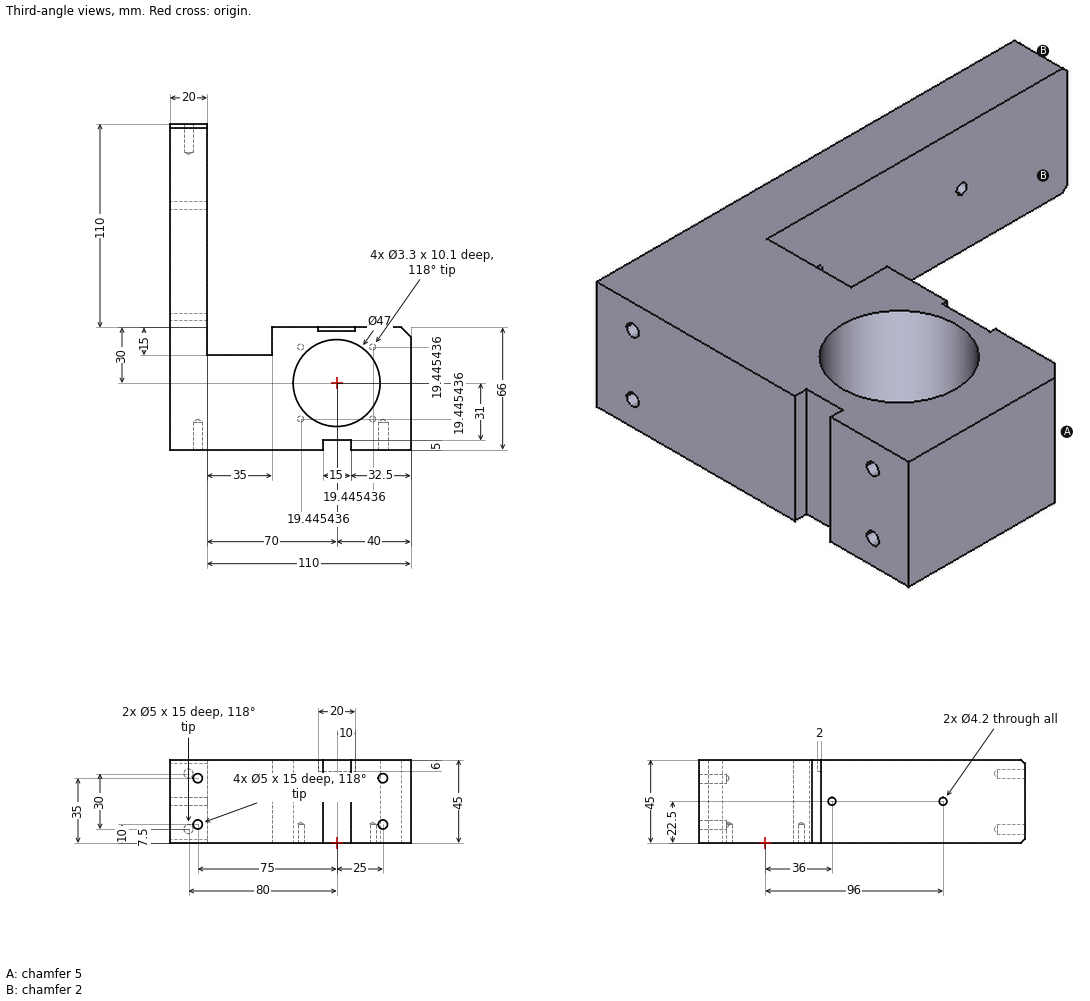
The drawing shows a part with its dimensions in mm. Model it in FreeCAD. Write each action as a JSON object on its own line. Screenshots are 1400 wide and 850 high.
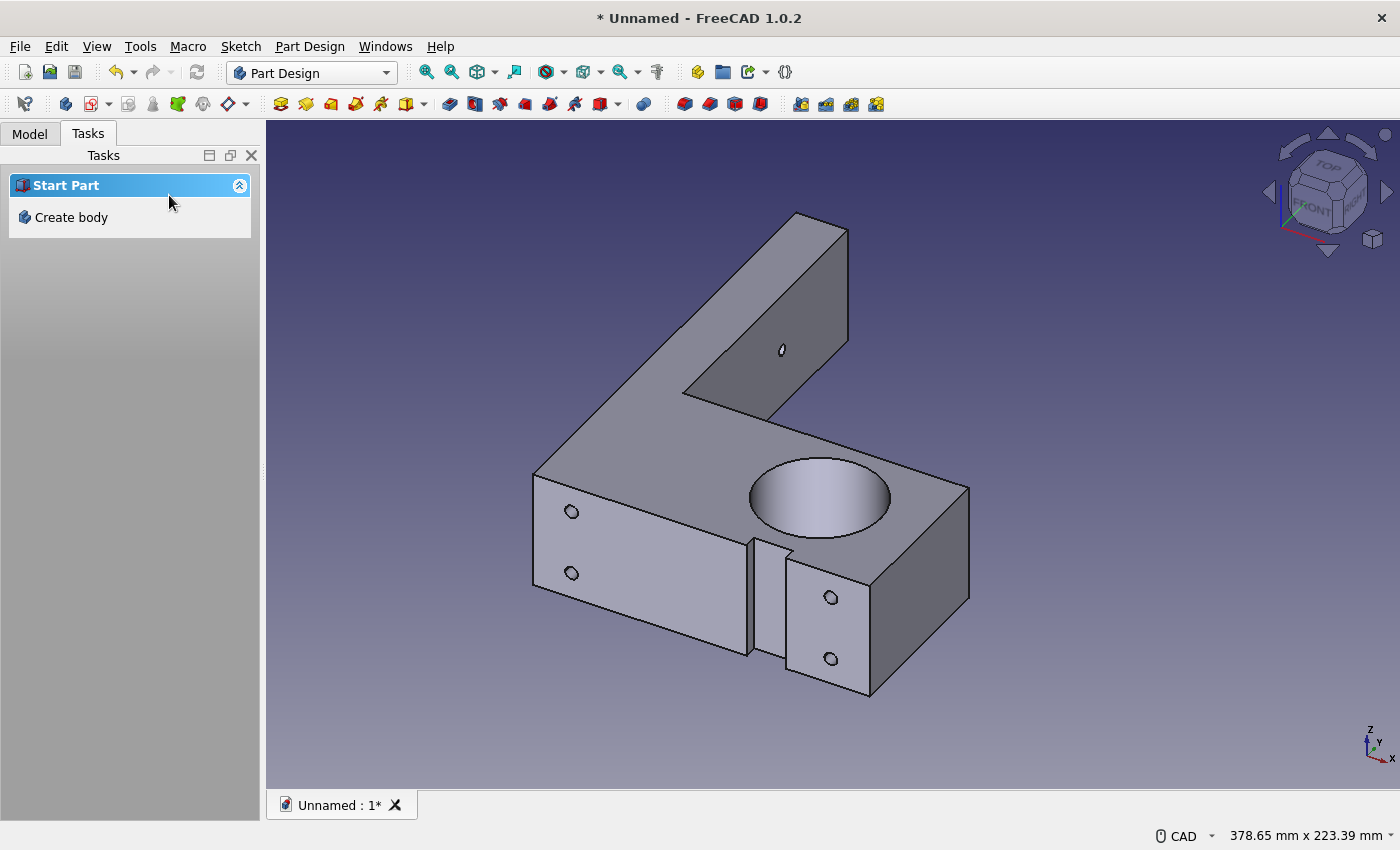
{"action": "key", "text": "4"}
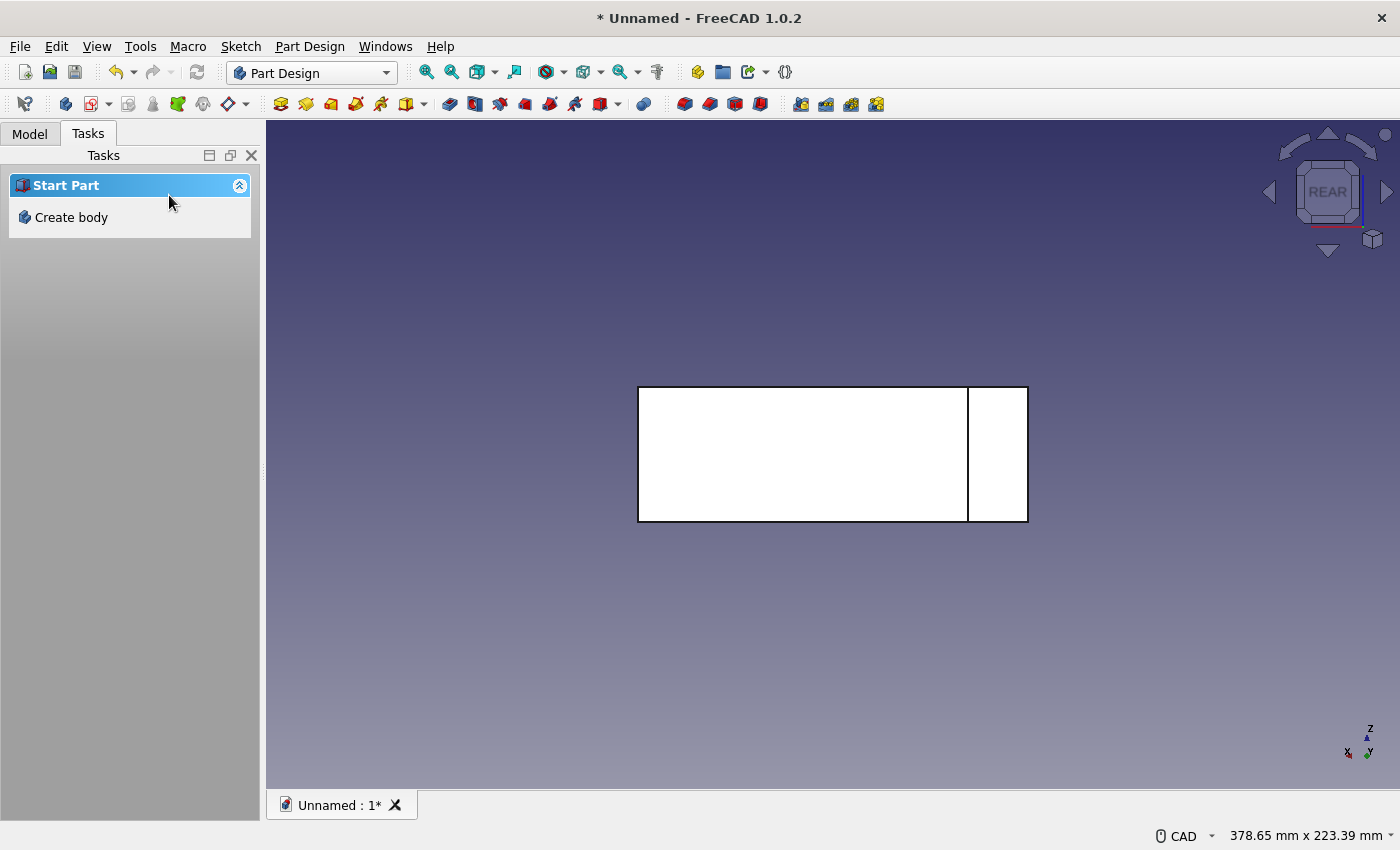
{"action": "key", "text": "v f"}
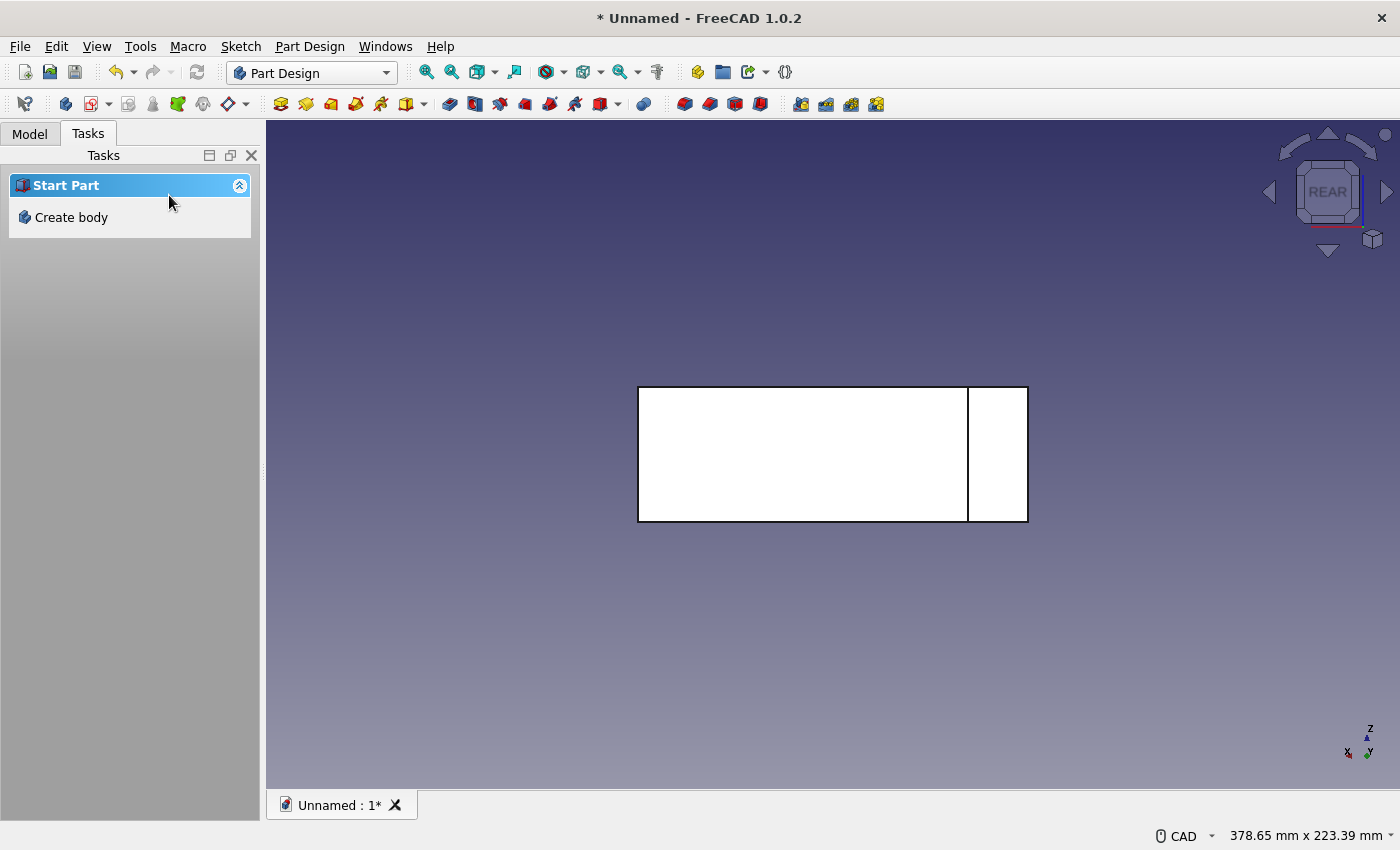
{"action": "left_click", "coordinate": [998, 434]}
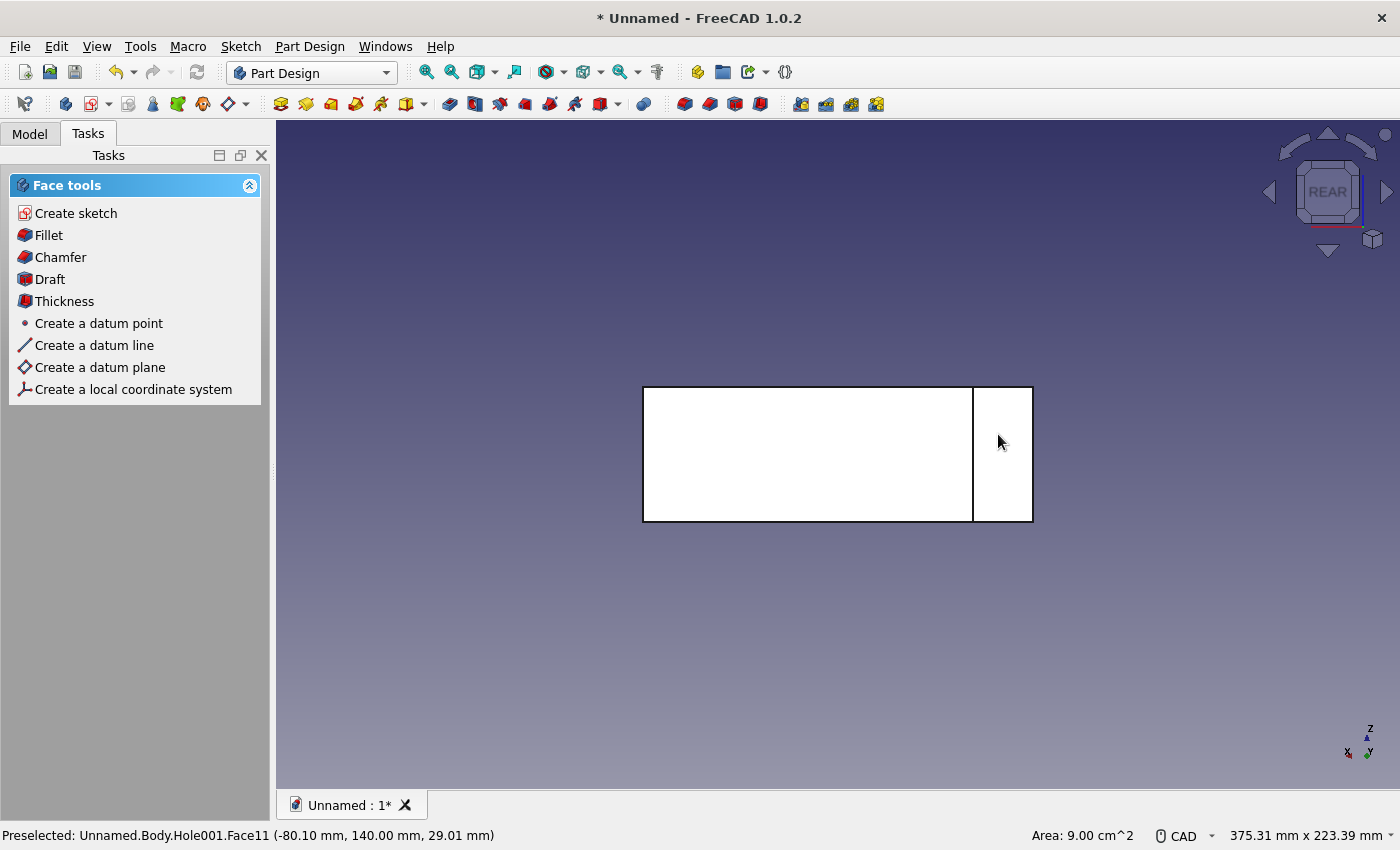
{"action": "left_click", "coordinate": [90, 104]}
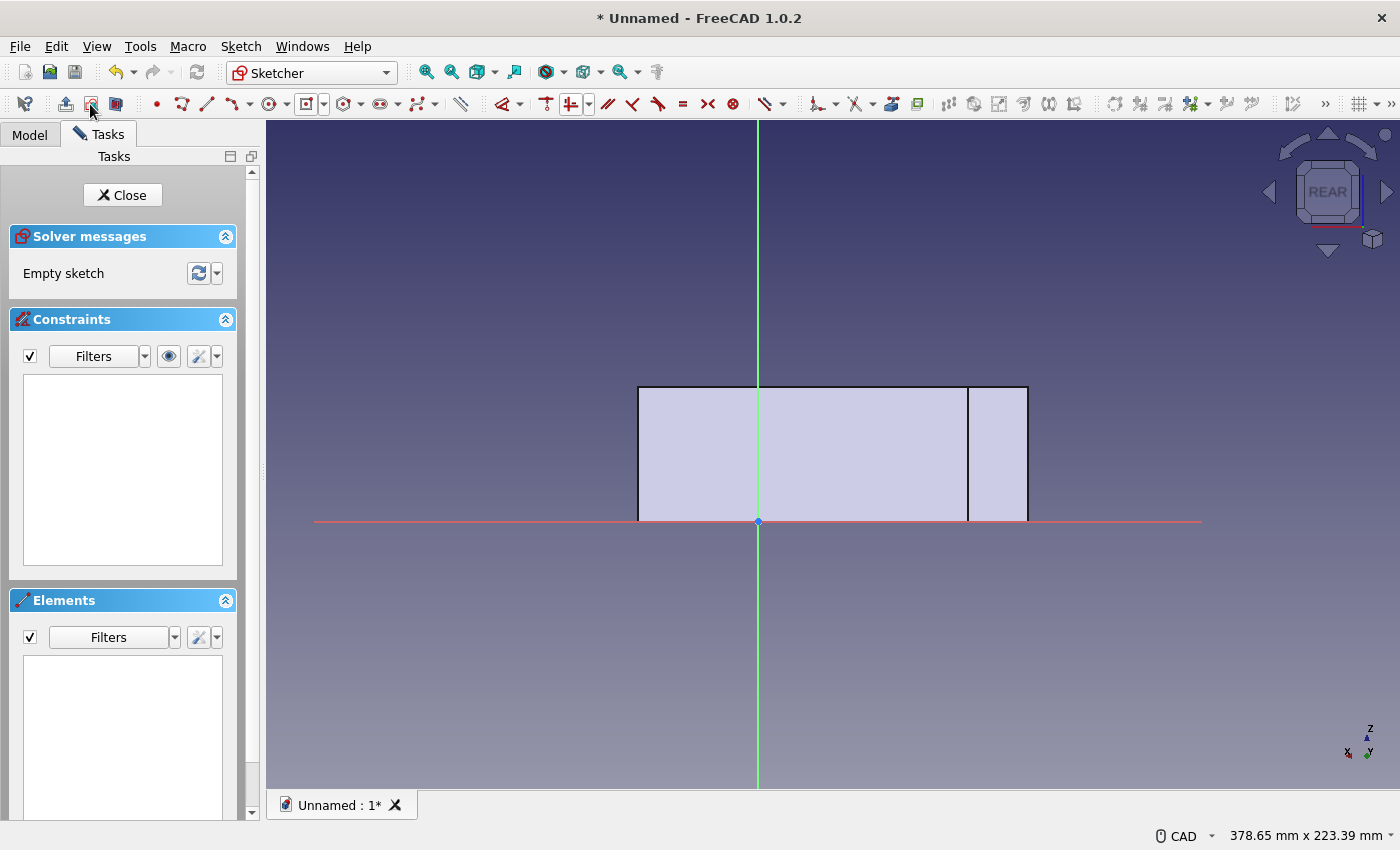
{"action": "scroll", "coordinate": [950, 466], "scroll_direction": "up", "scroll_amount": 5}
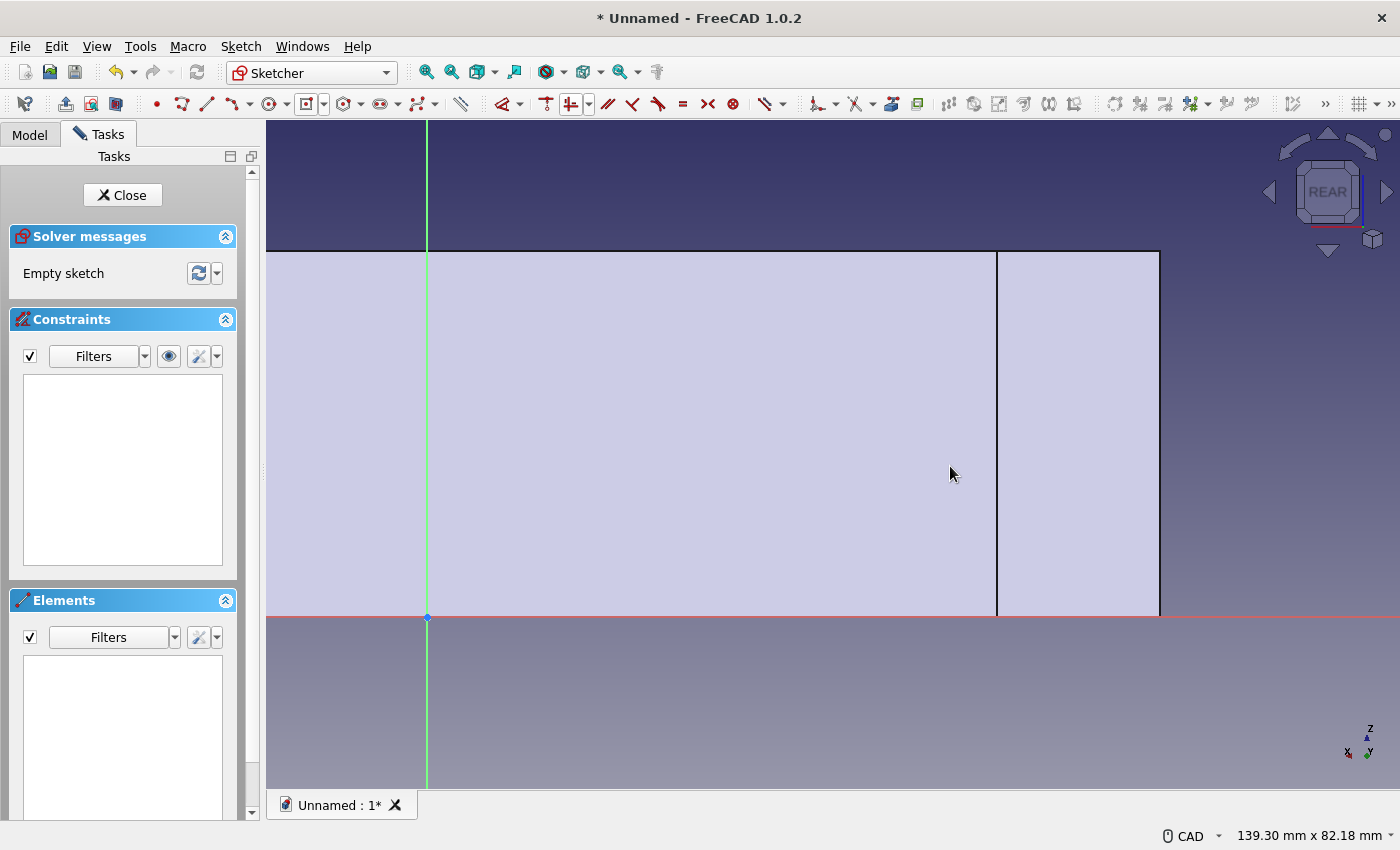
{"action": "left_click", "coordinate": [268, 104]}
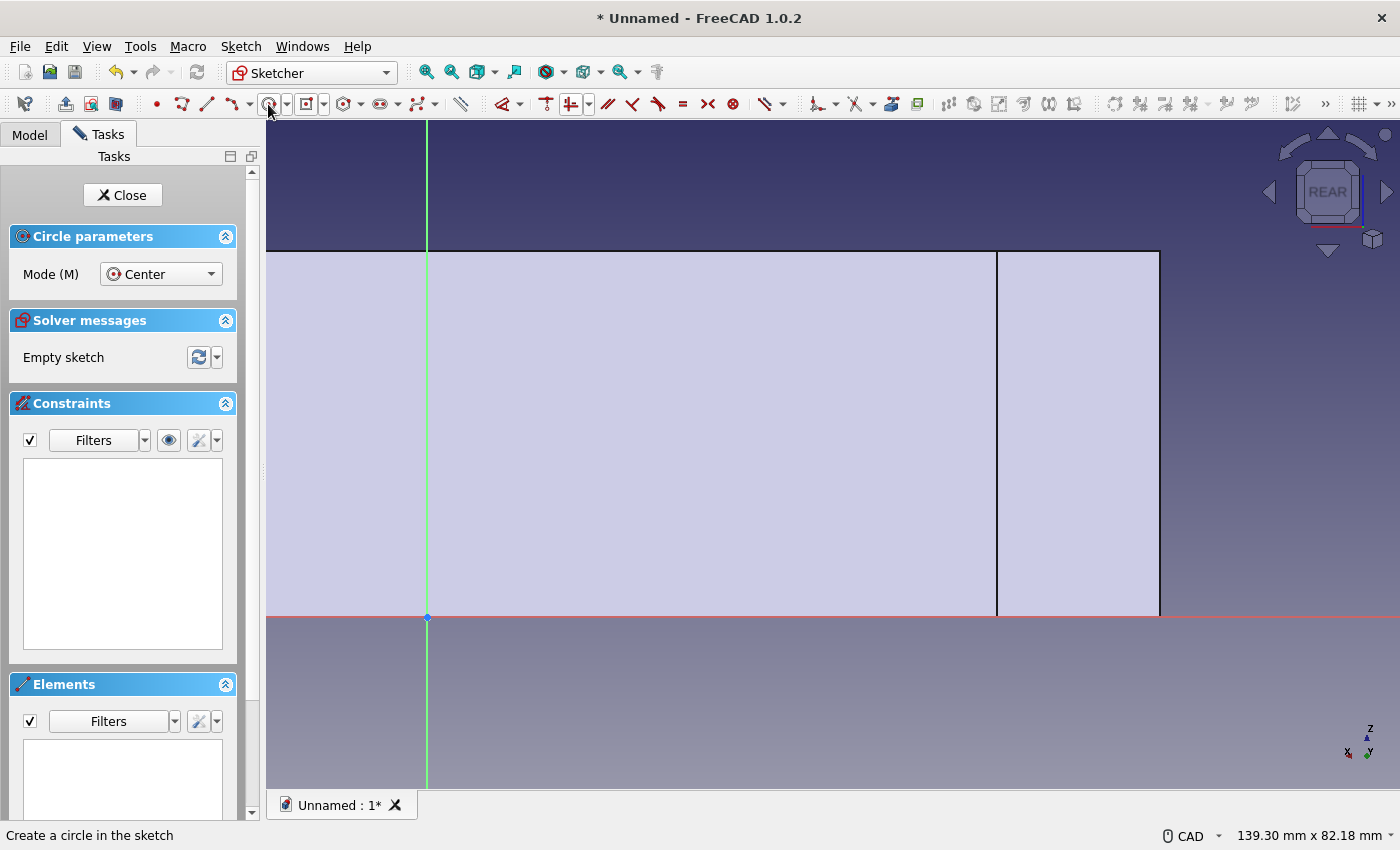
{"action": "left_click", "coordinate": [1079, 556]}
{"action": "left_click", "coordinate": [1093, 542]}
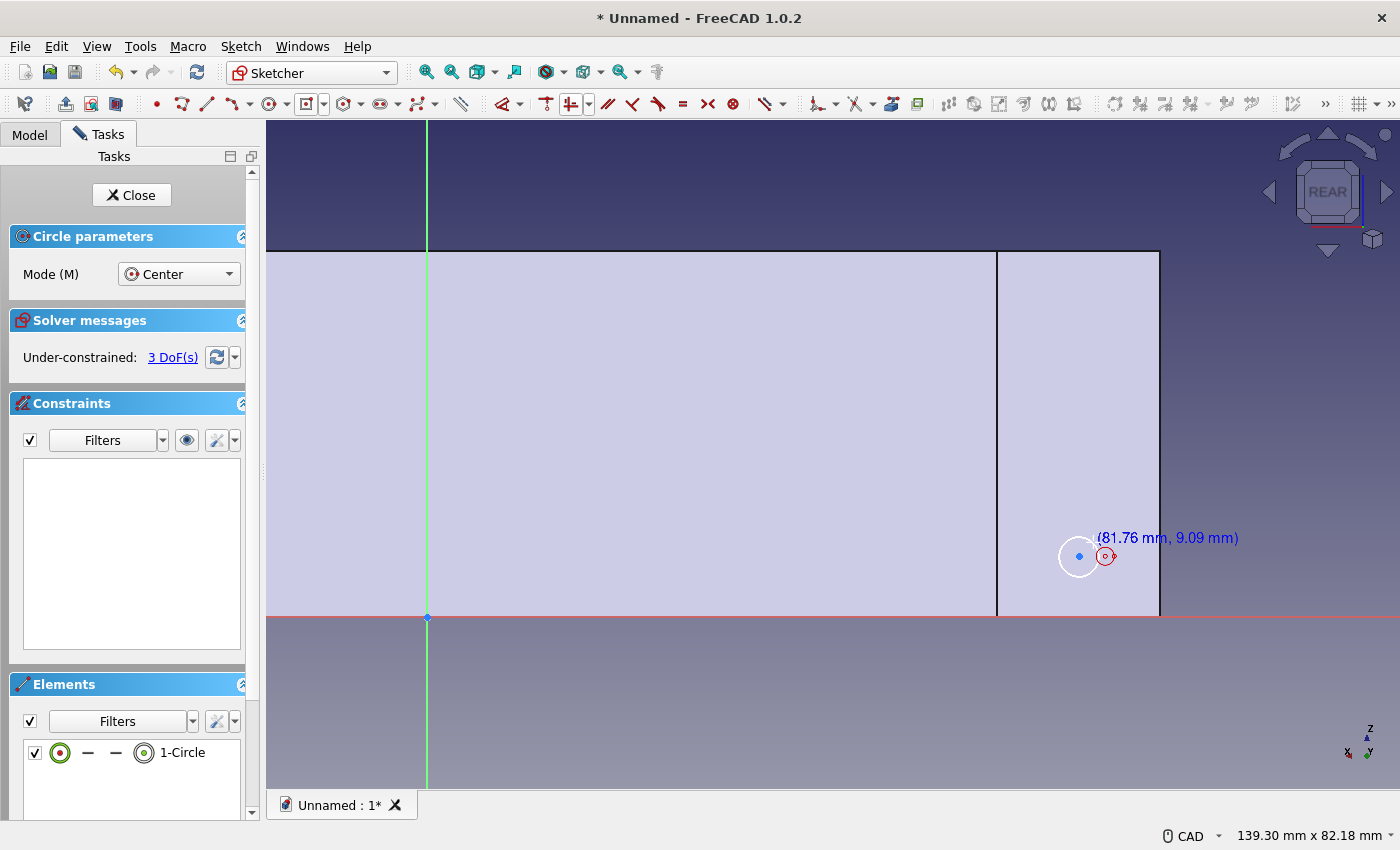
{"action": "left_click", "coordinate": [1079, 312]}
{"action": "left_click", "coordinate": [1093, 297]}
{"action": "key", "text": "Escape"}